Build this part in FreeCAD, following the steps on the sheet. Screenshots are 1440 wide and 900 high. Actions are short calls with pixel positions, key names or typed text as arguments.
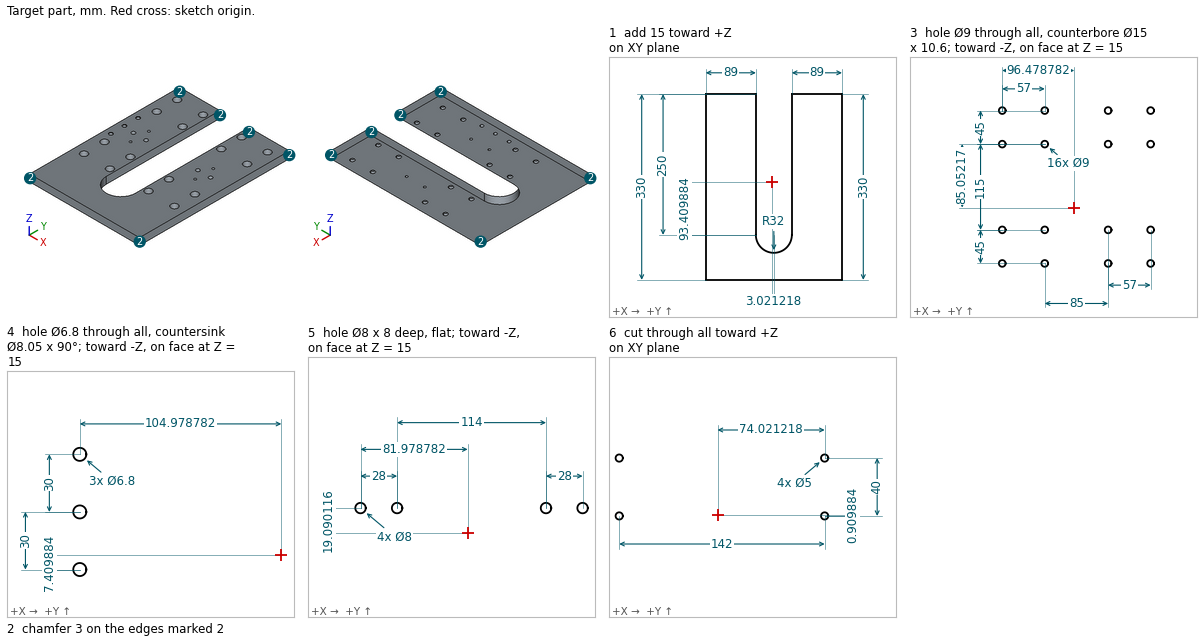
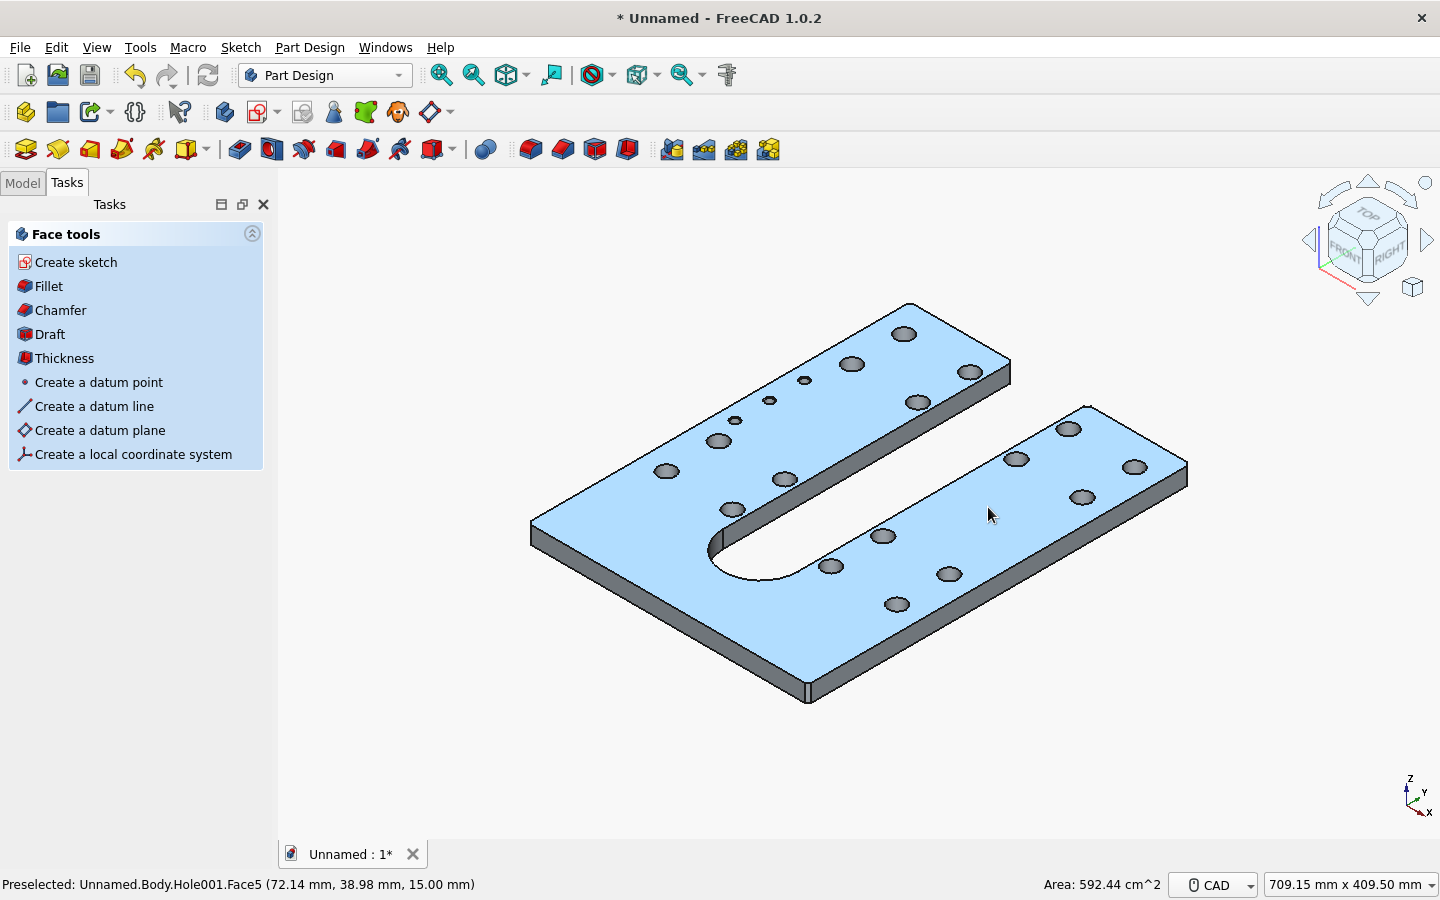
click(258, 112)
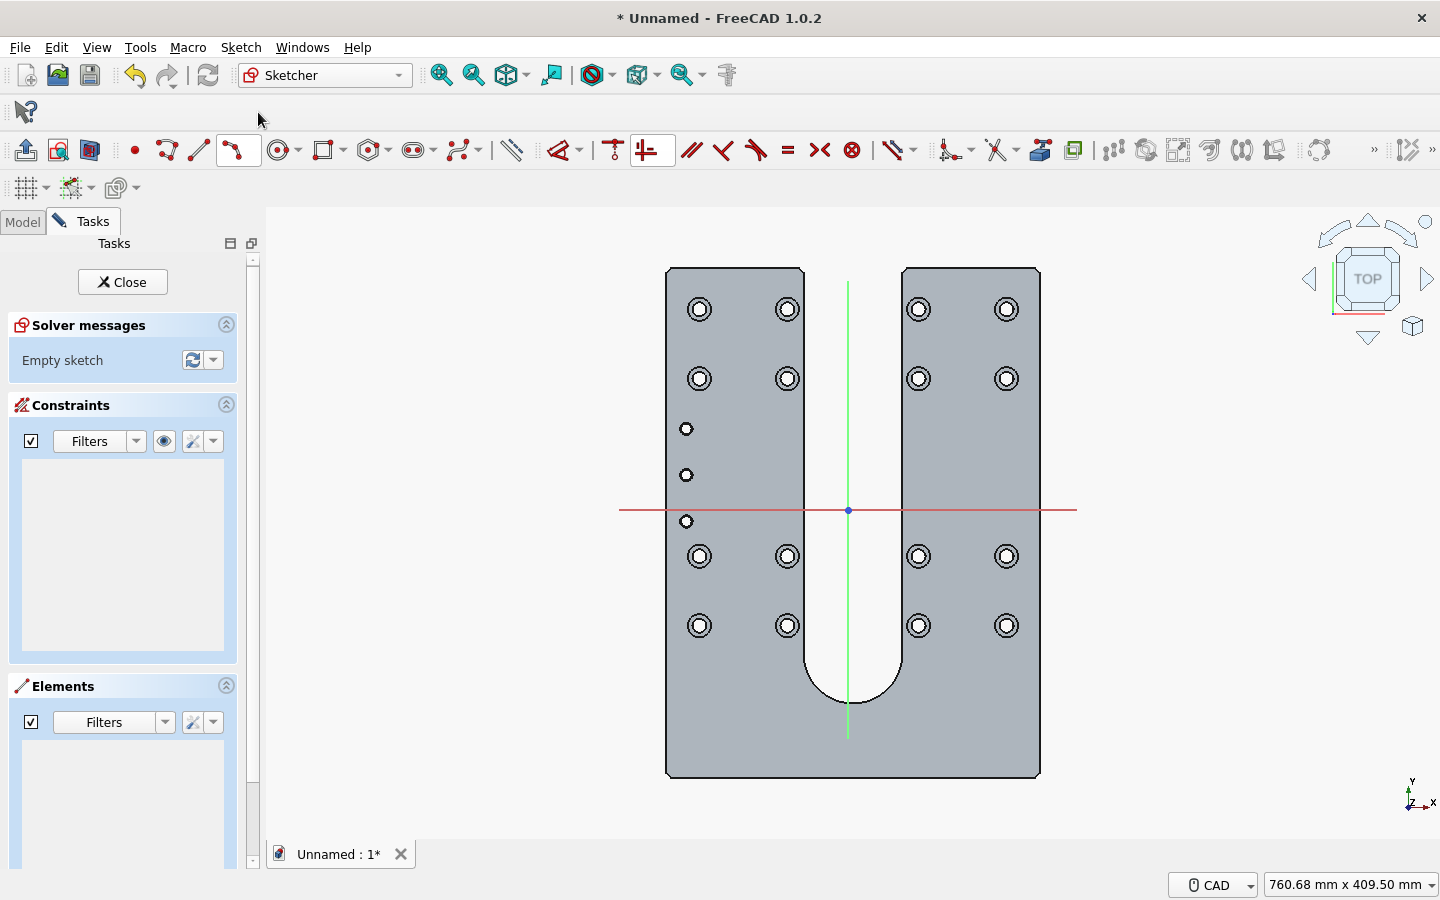
scroll(893, 474, up, 5)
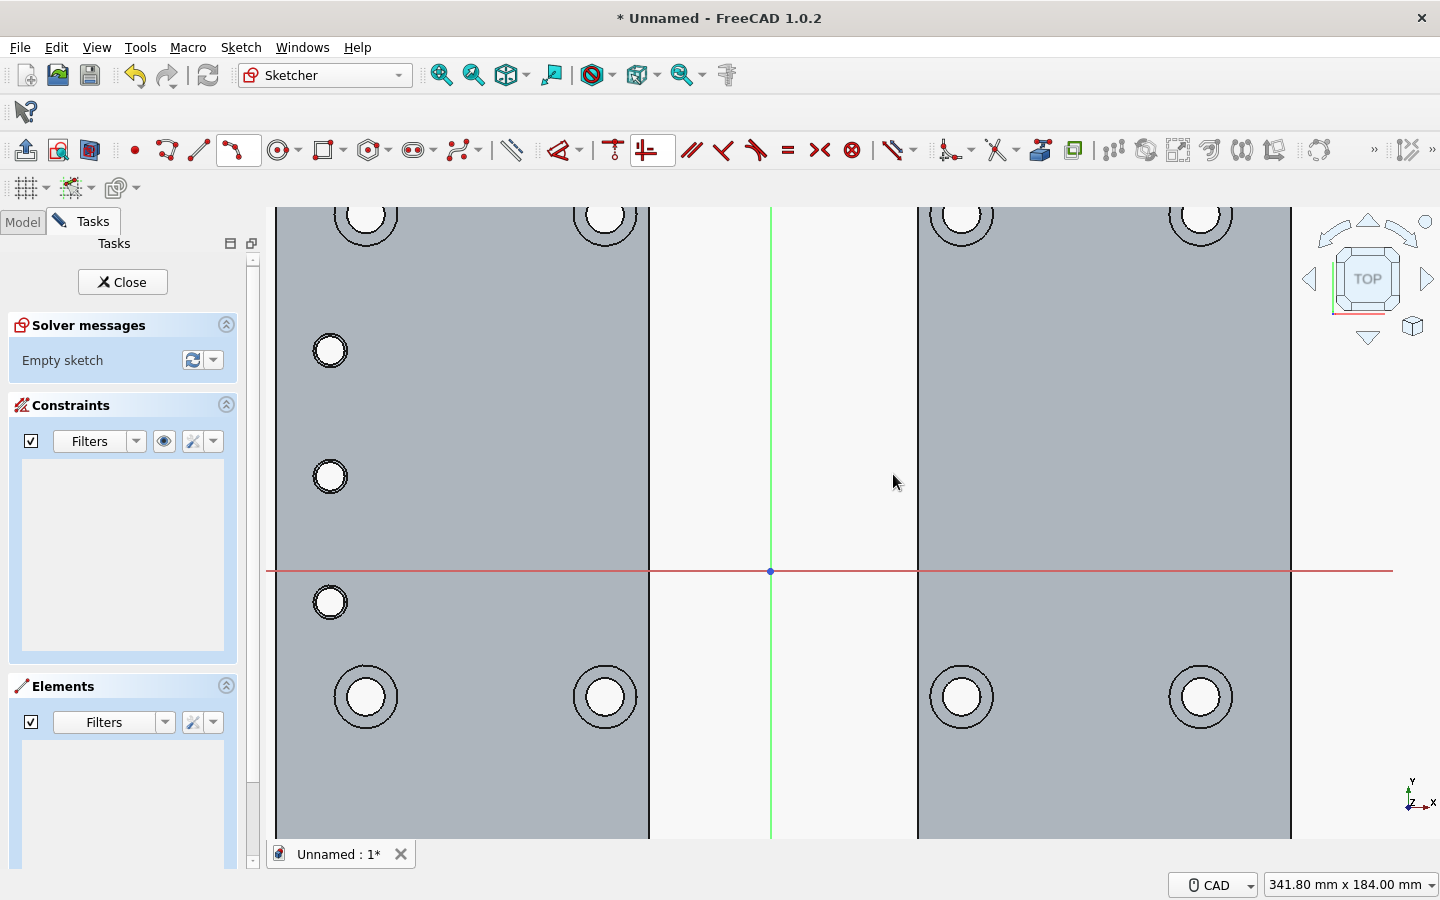
click(278, 150)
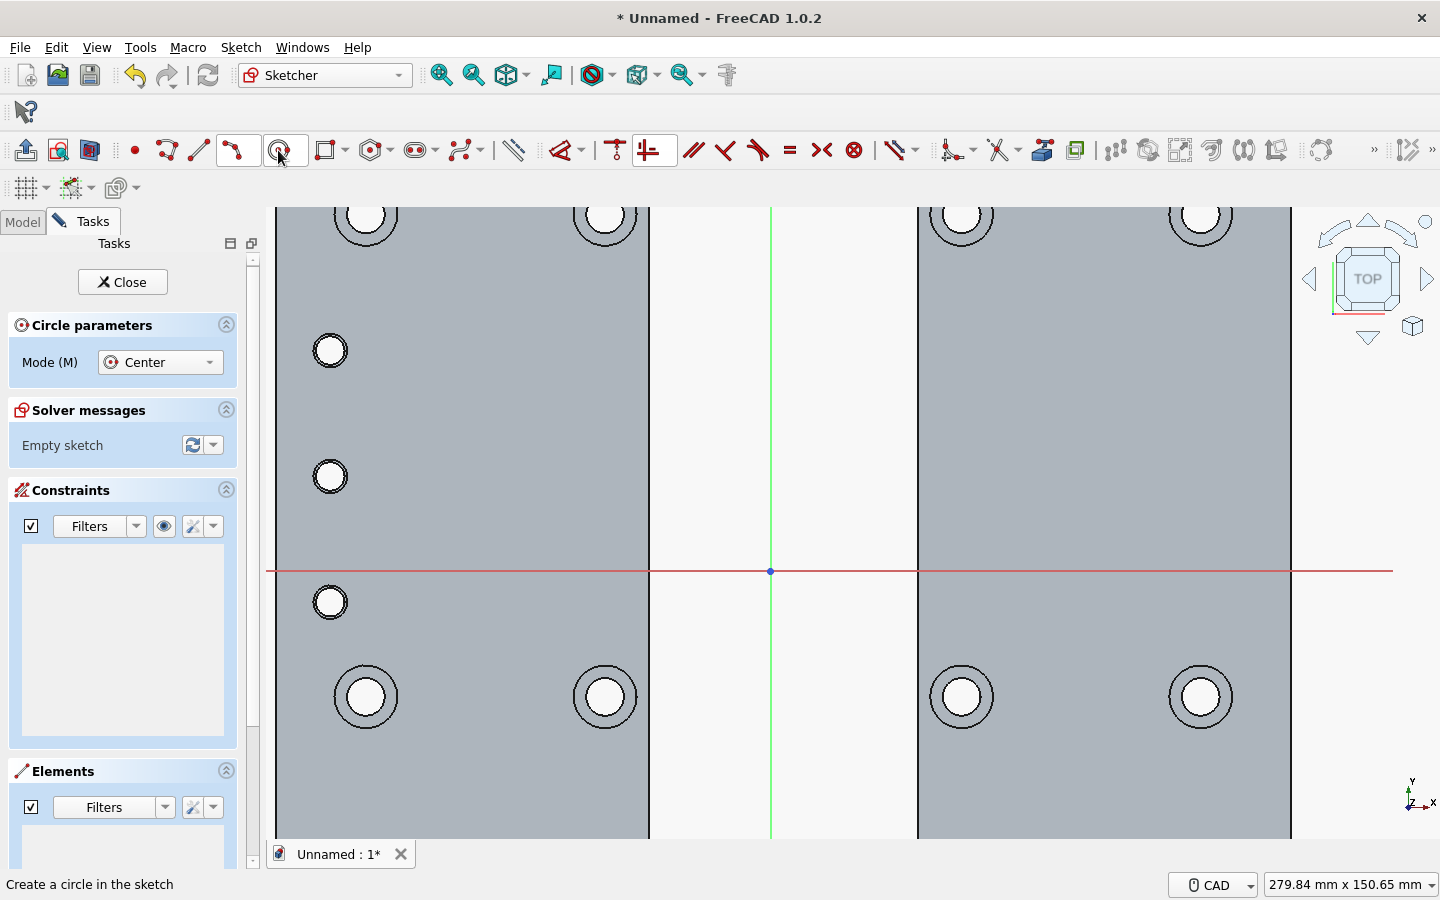
scroll(427, 491, up, 2)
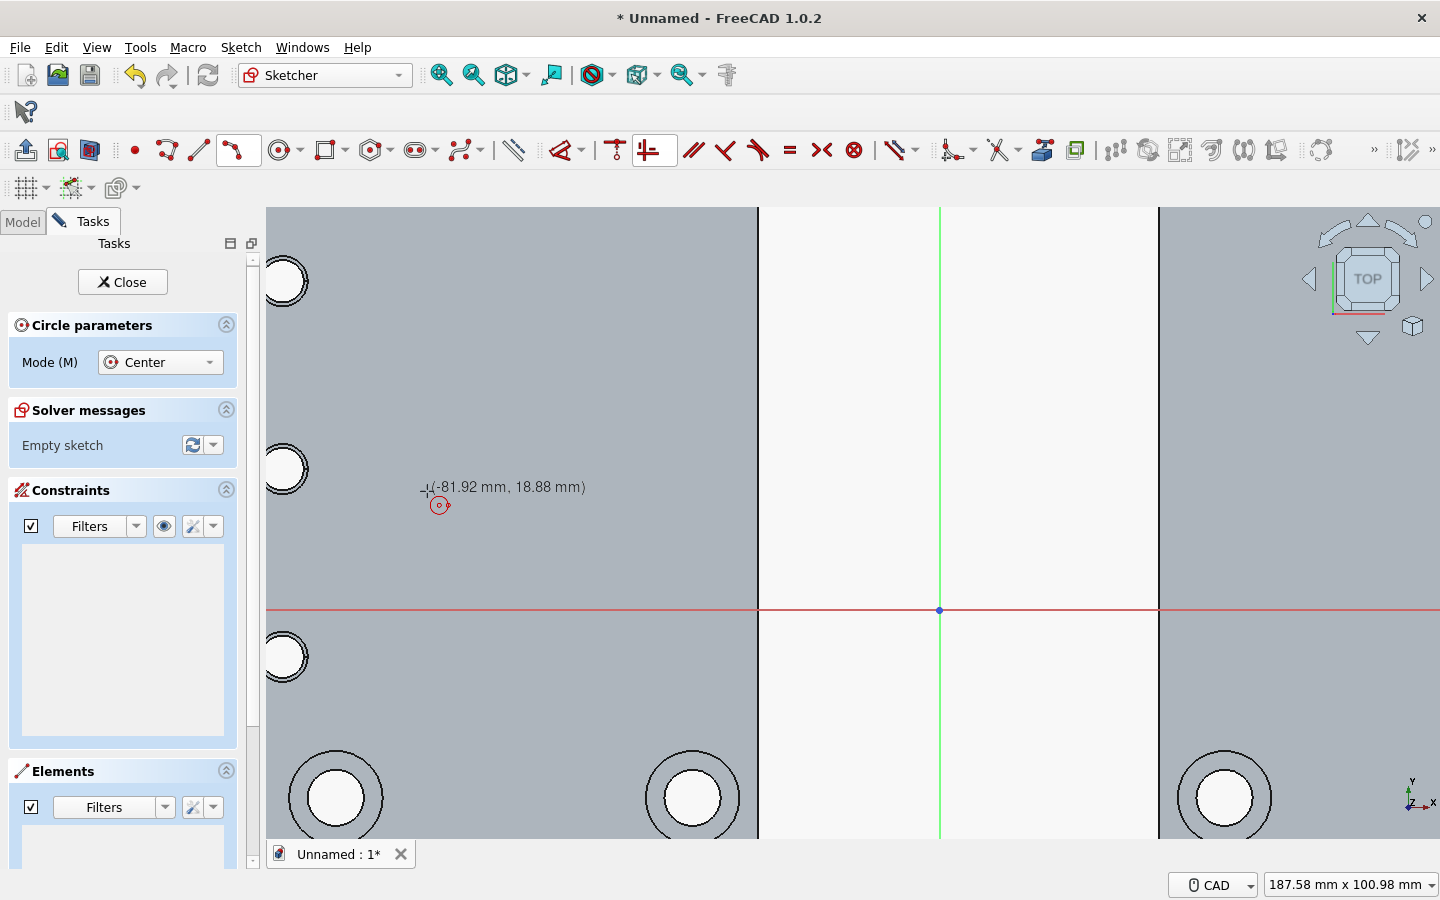
click(427, 491)
move(444, 473)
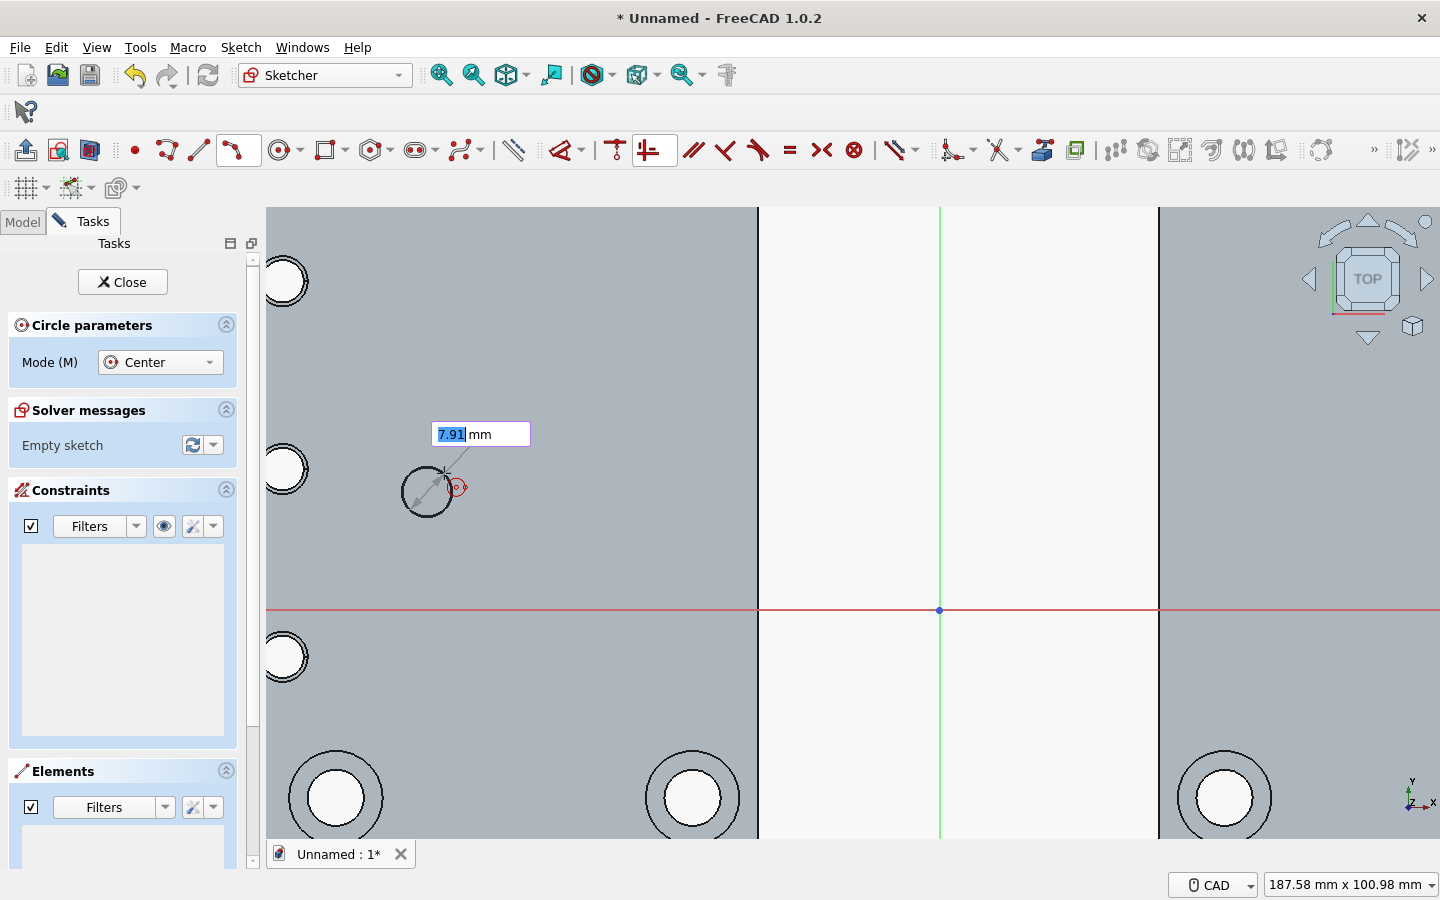
text(8)
key(Return)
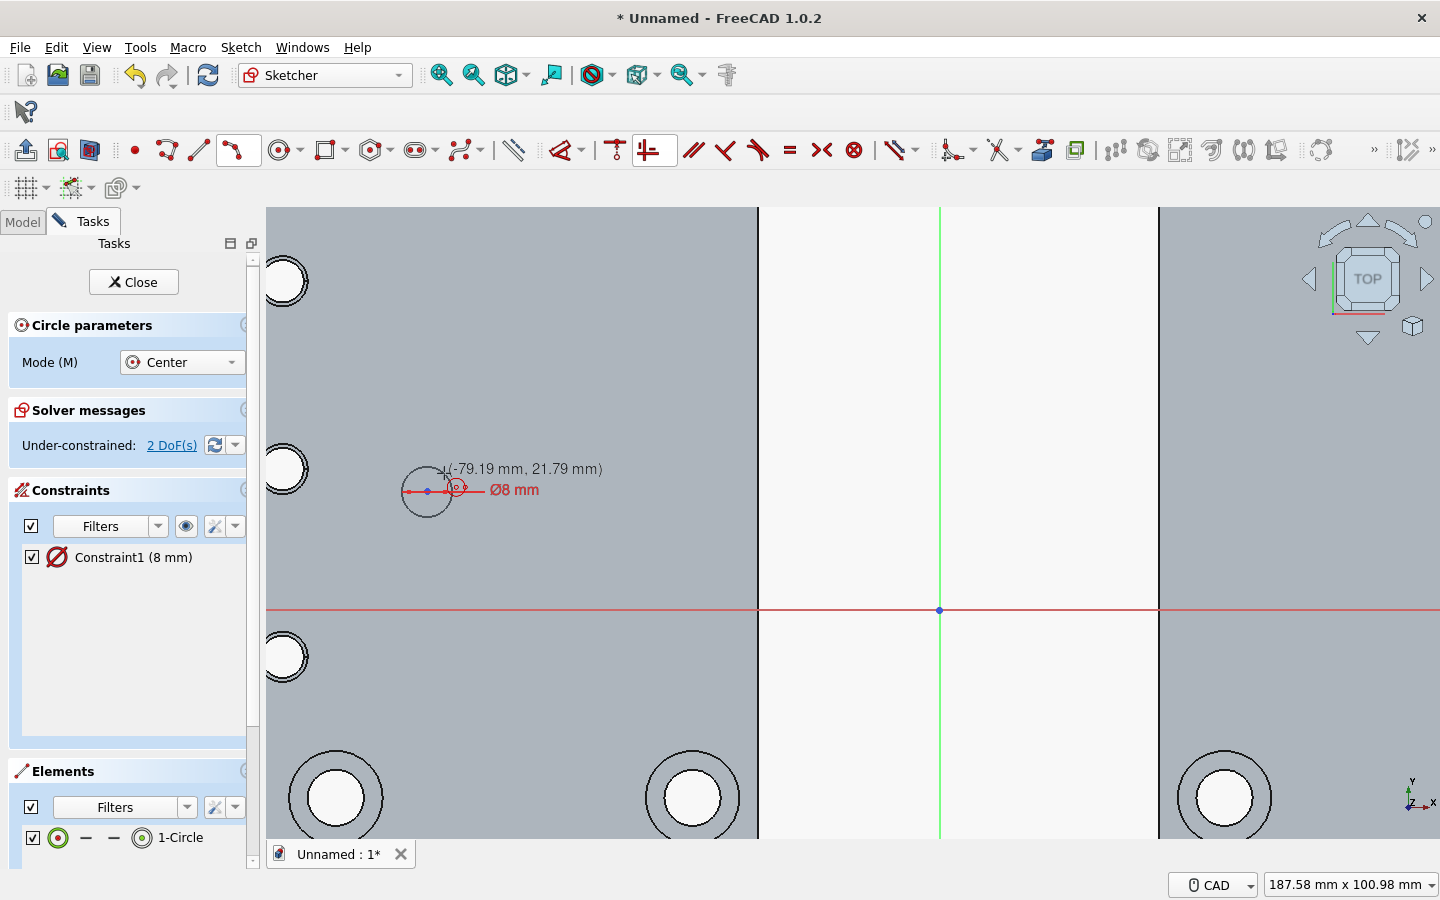
click(602, 491)
move(620, 473)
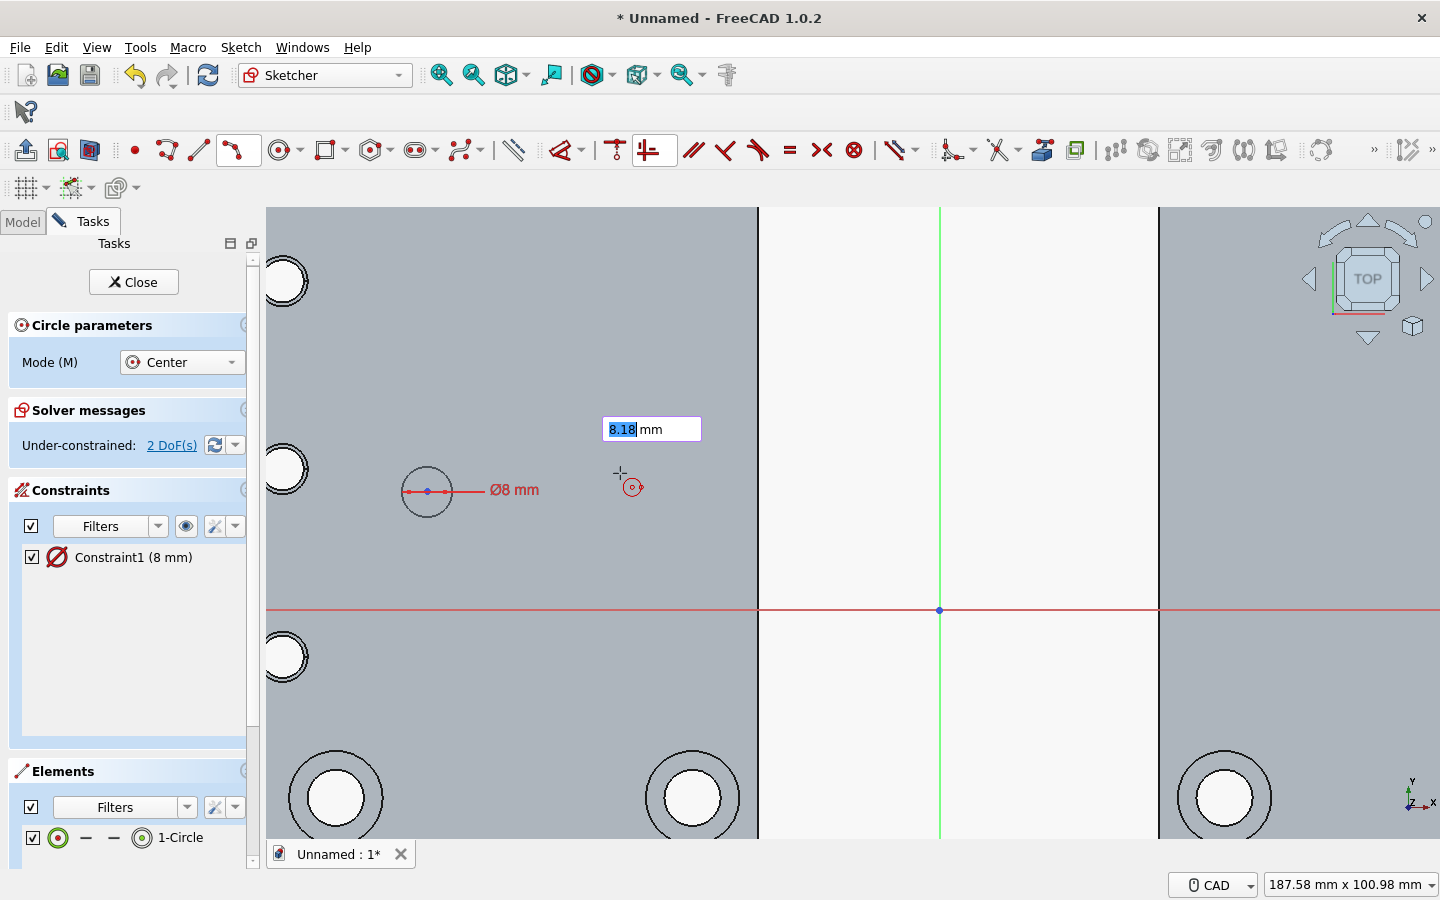
text(8)
key(Return)